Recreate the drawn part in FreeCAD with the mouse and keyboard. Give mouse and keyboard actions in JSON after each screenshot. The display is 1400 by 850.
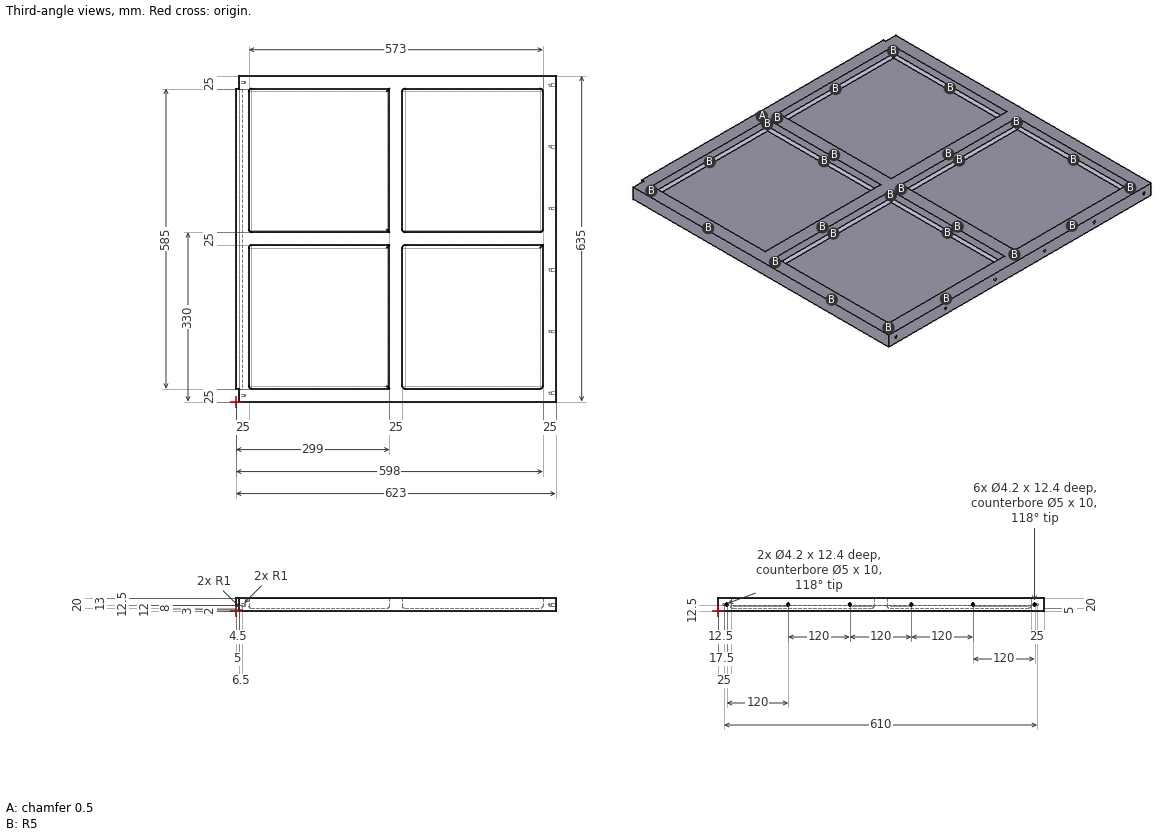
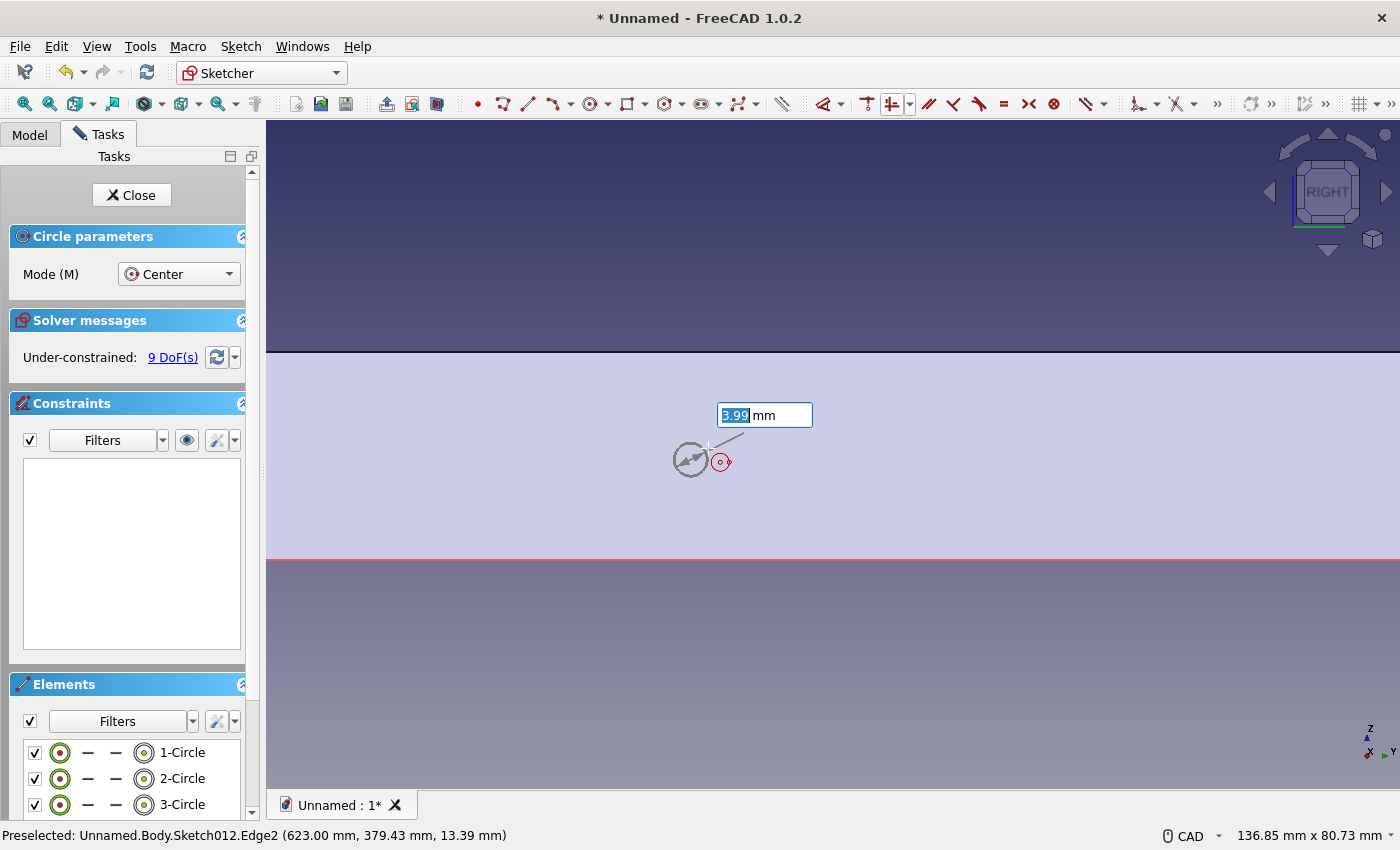
{"action": "left_click", "coordinate": [705, 444]}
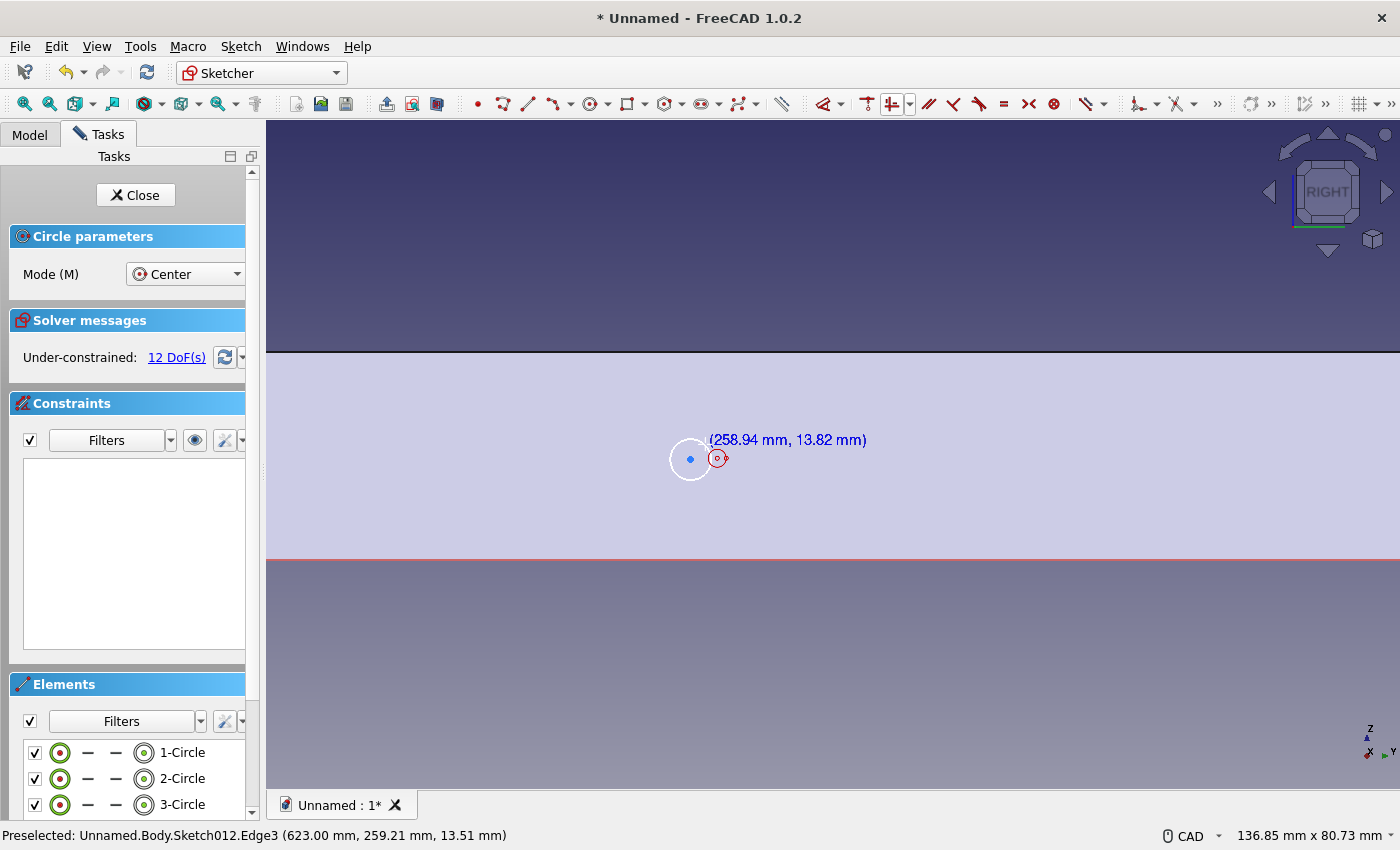
{"action": "scroll", "coordinate": [708, 448], "scroll_direction": "down", "scroll_amount": 10}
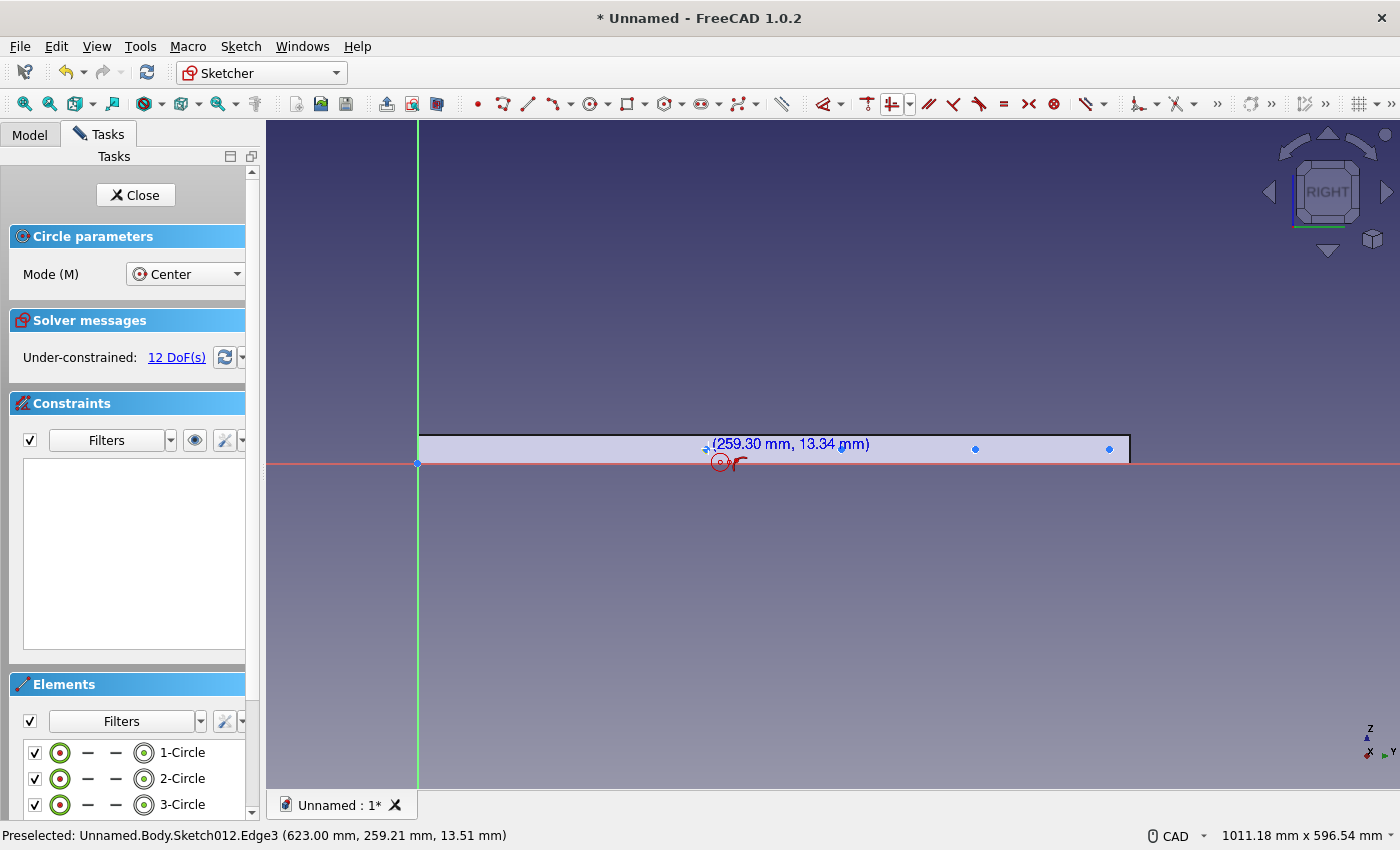
{"action": "scroll", "coordinate": [572, 449], "scroll_direction": "up", "scroll_amount": 12}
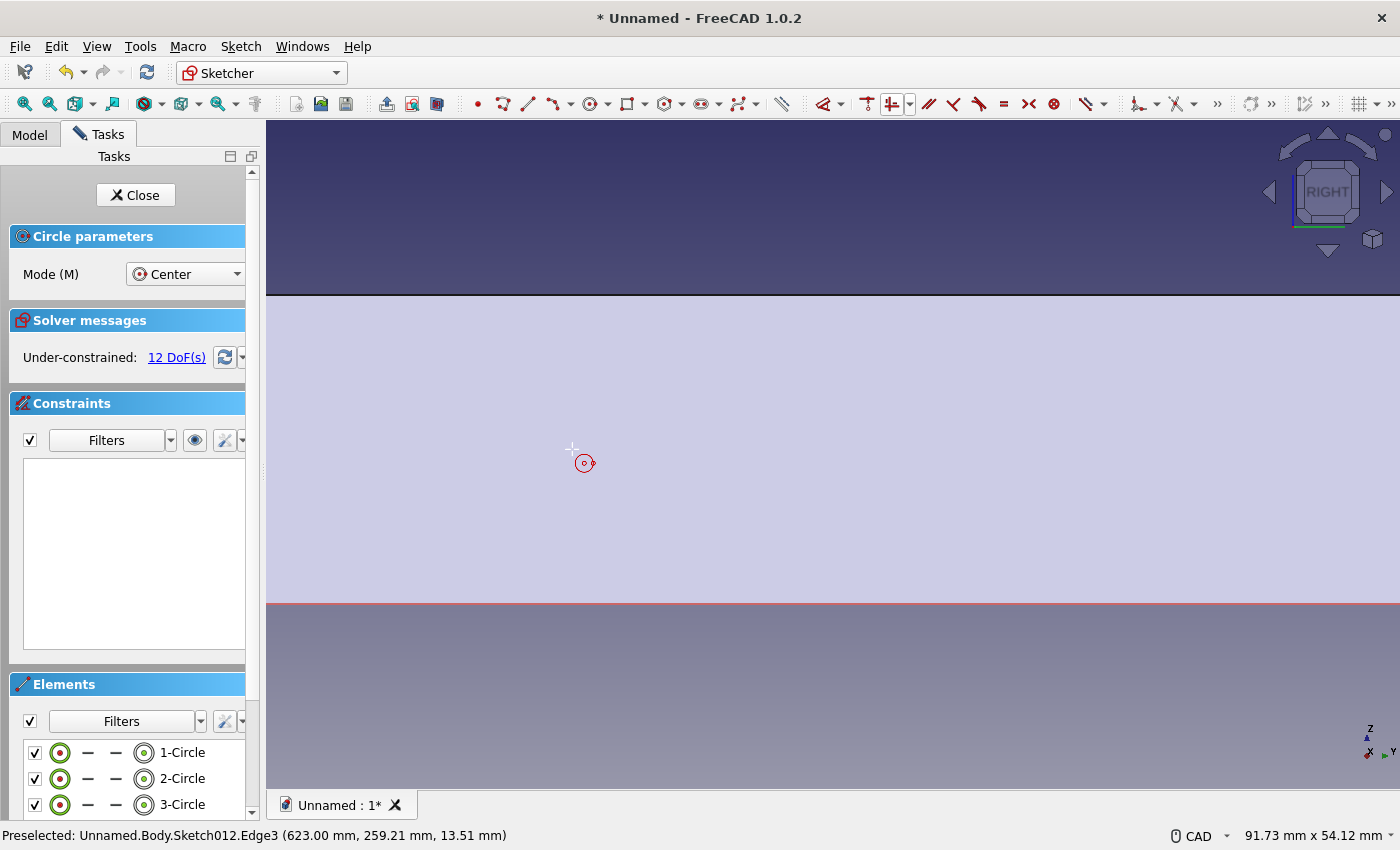
{"action": "scroll", "coordinate": [572, 449], "scroll_direction": "down", "scroll_amount": 12}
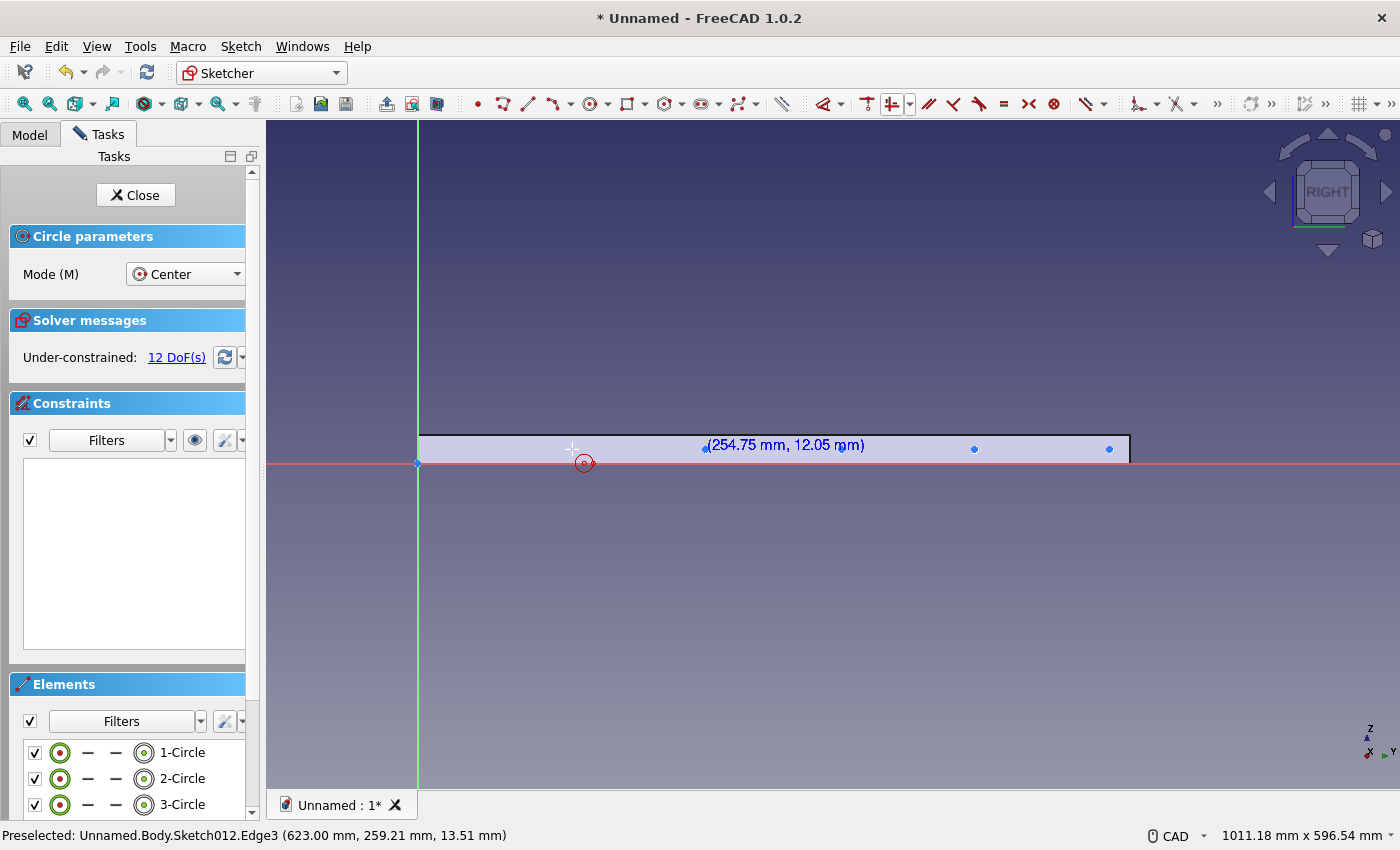
{"action": "left_click", "coordinate": [572, 449]}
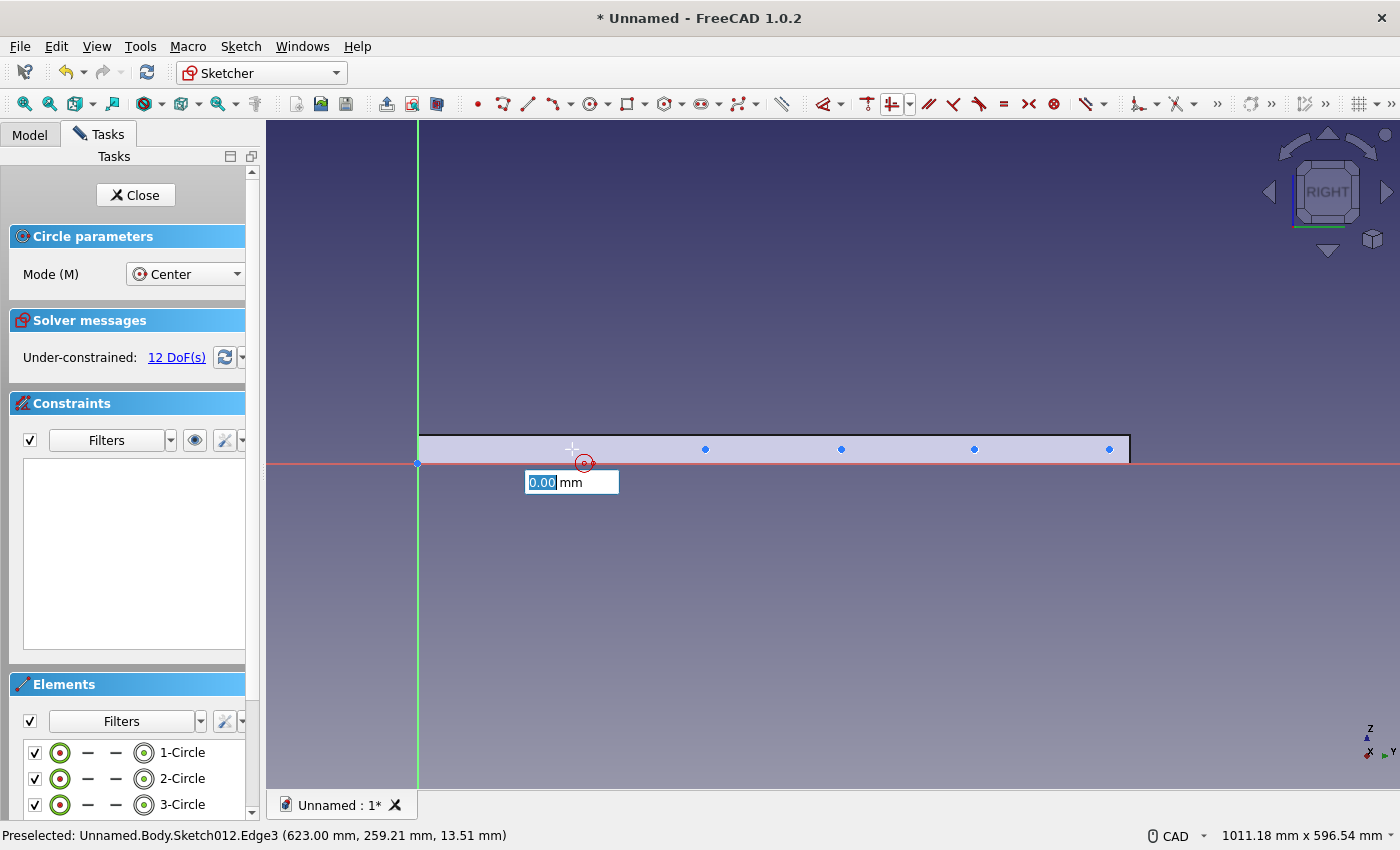
{"action": "scroll", "coordinate": [573, 448], "scroll_direction": "up", "scroll_amount": 10}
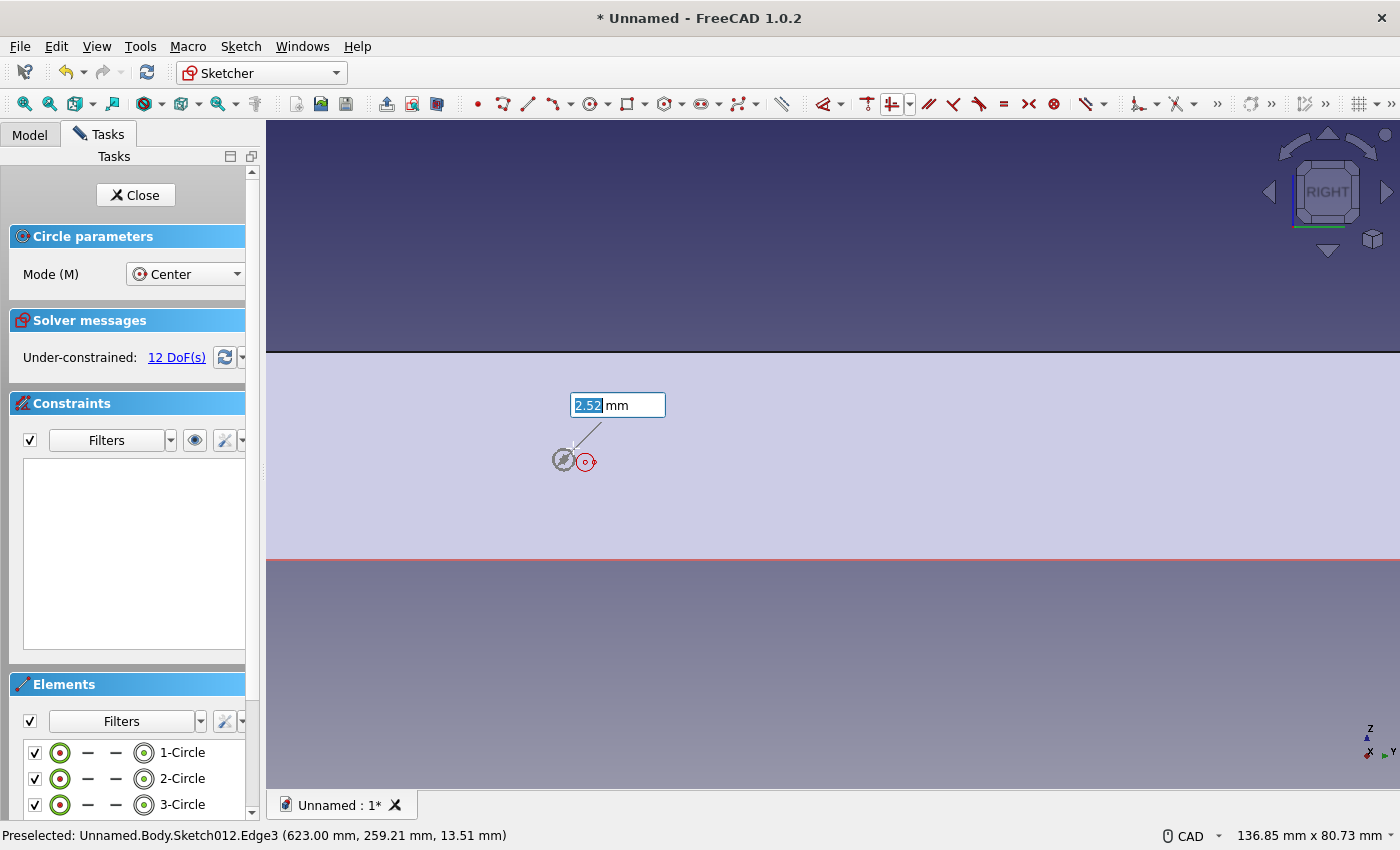
{"action": "left_click", "coordinate": [574, 444]}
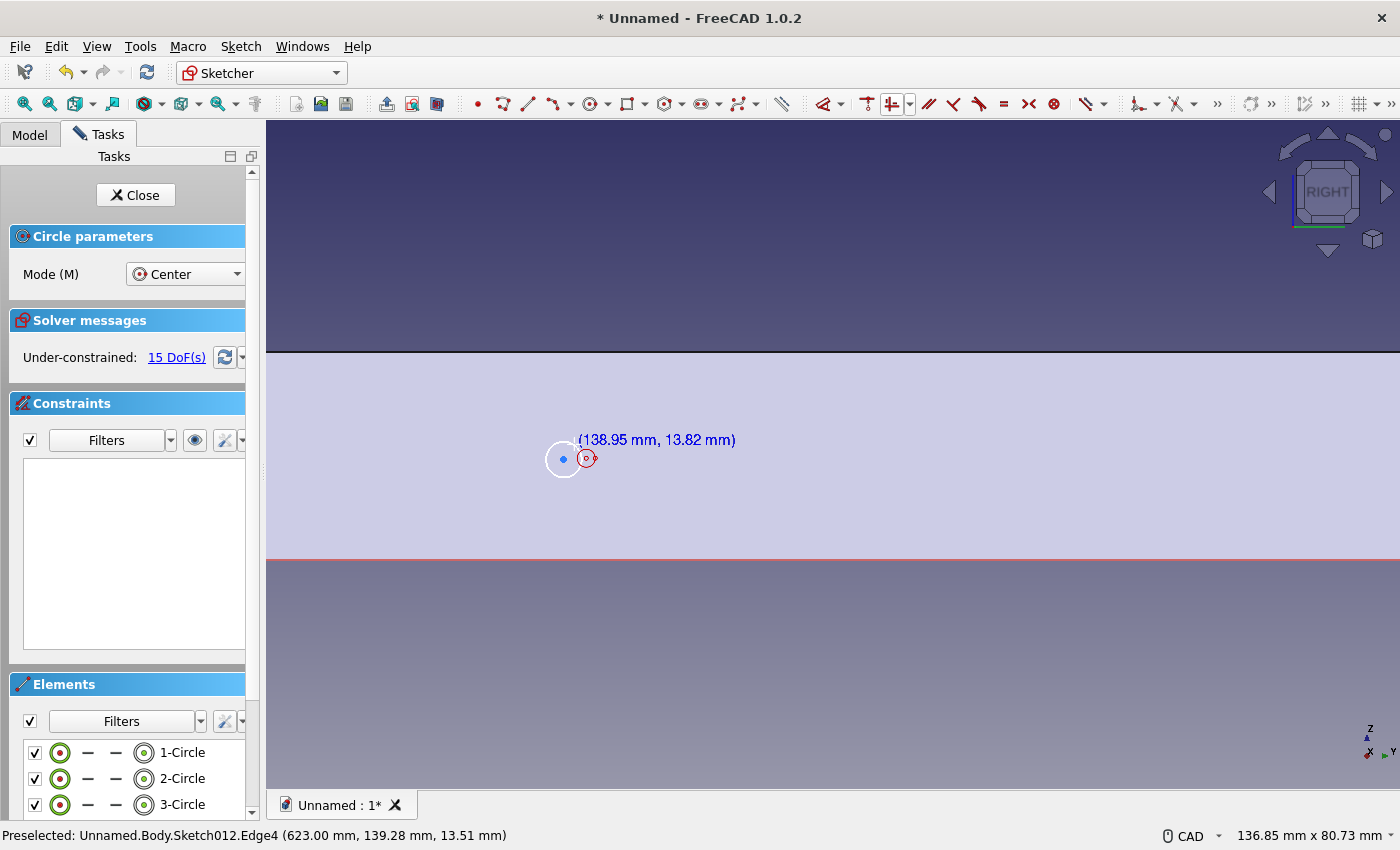
{"action": "scroll", "coordinate": [573, 448], "scroll_direction": "down", "scroll_amount": 10}